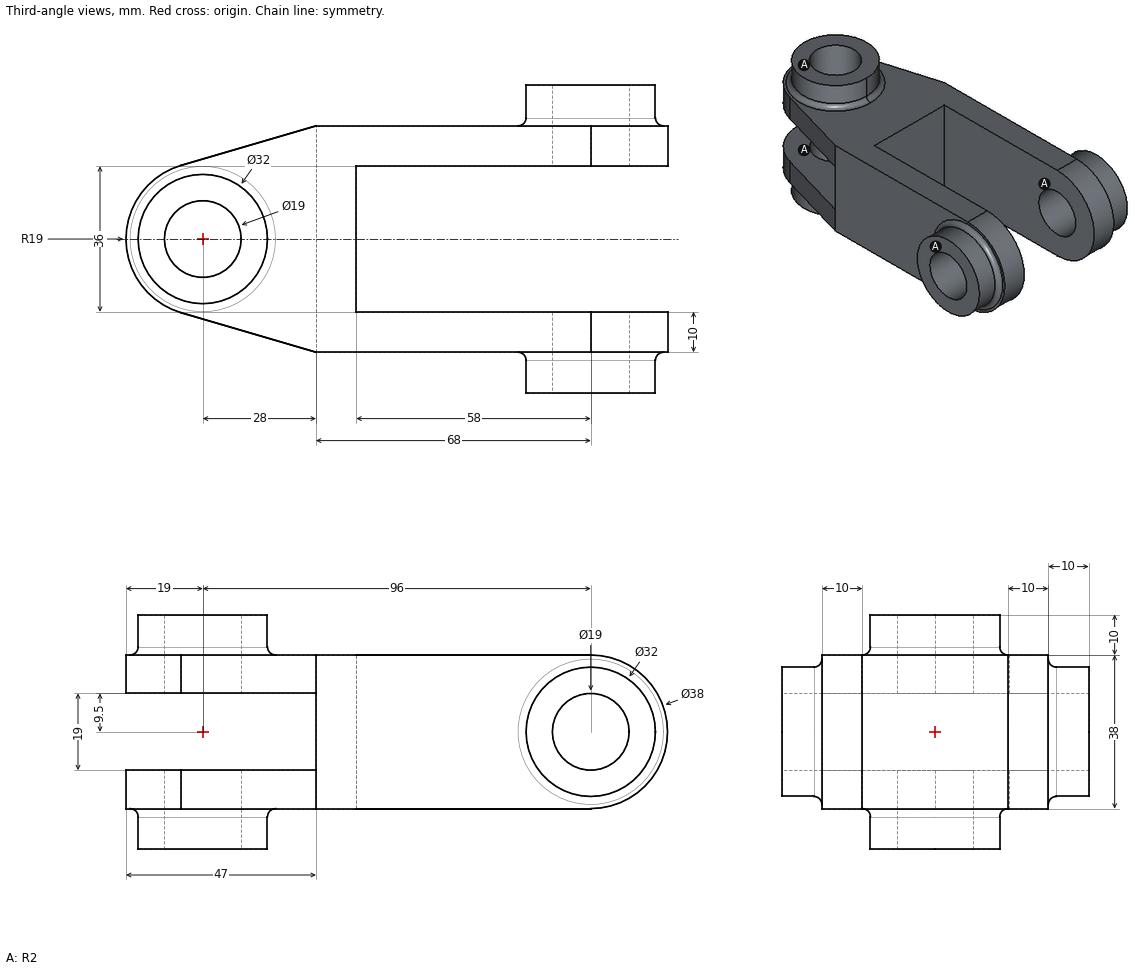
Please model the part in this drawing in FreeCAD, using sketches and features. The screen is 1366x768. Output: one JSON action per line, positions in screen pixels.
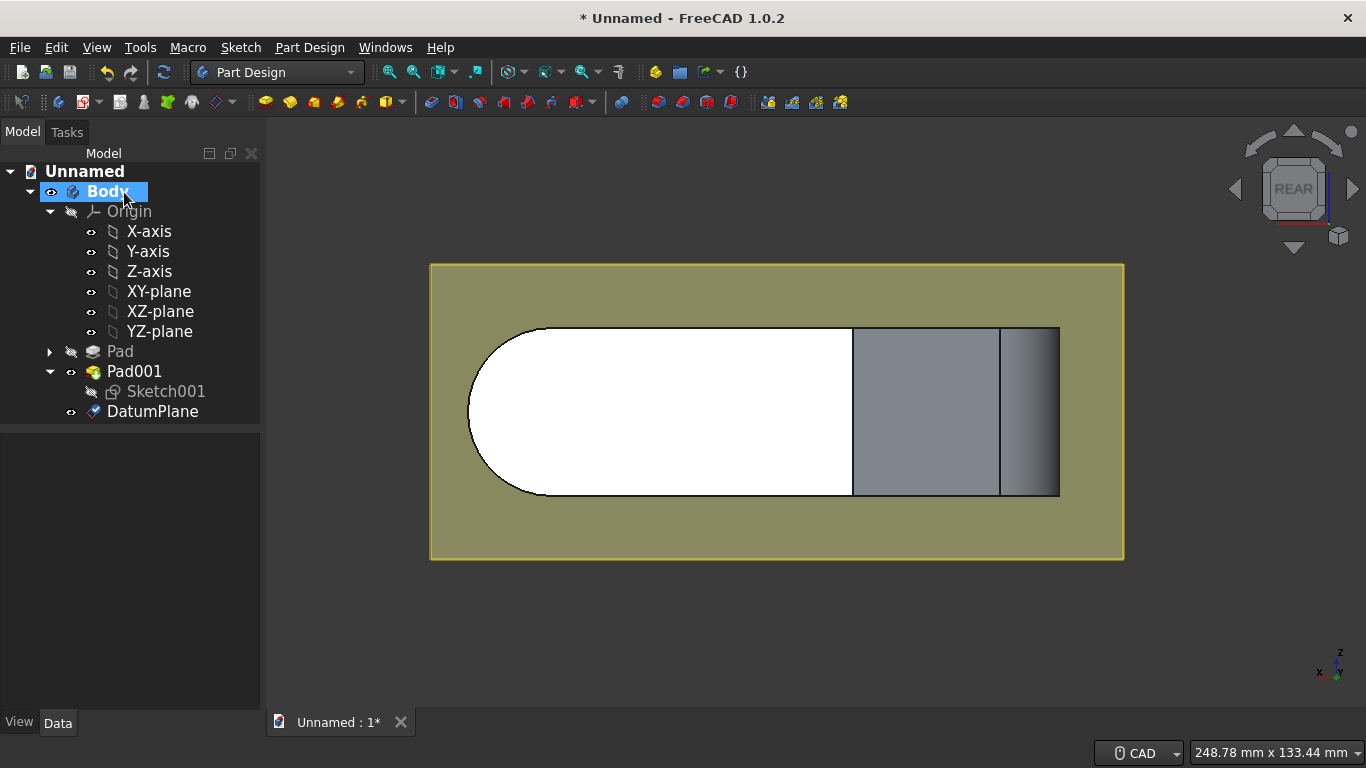
{"action": "left_click", "coordinate": [116, 412]}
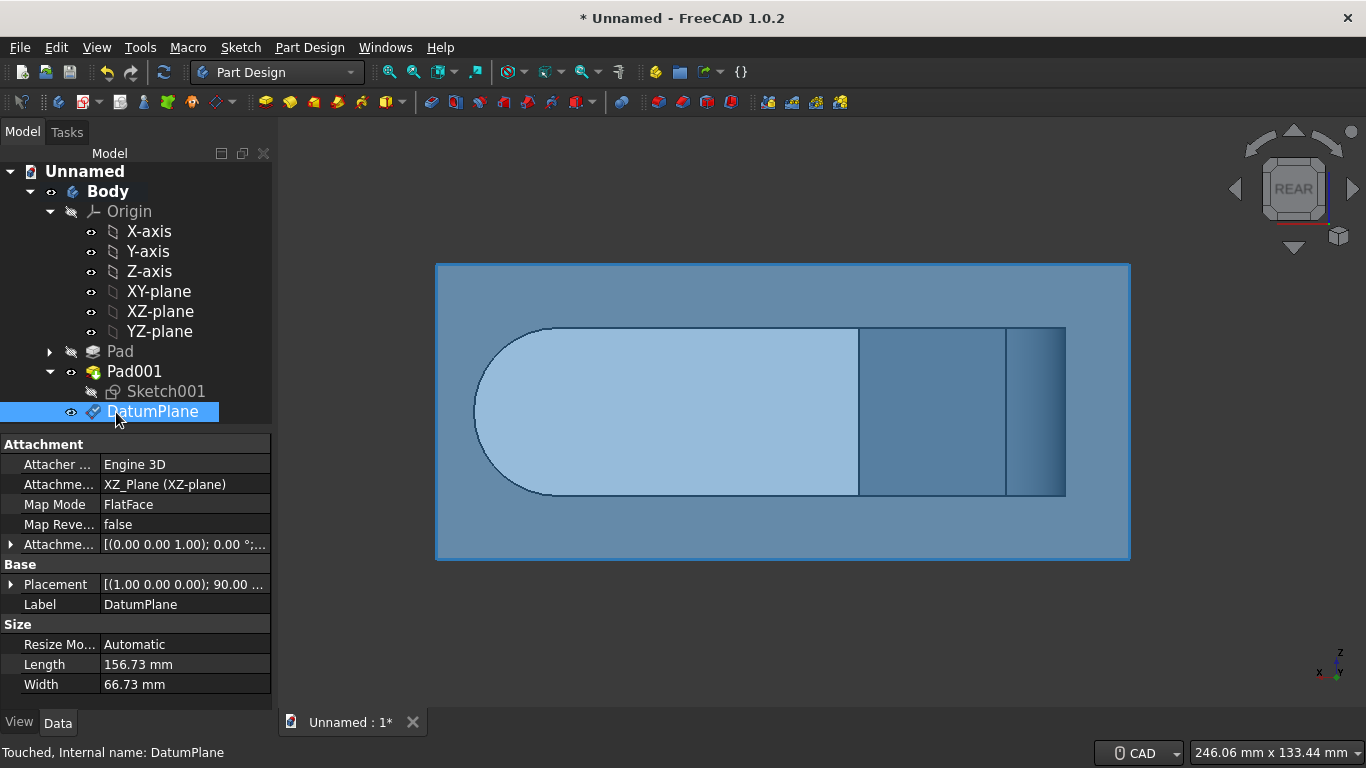
{"action": "left_click", "coordinate": [84, 102]}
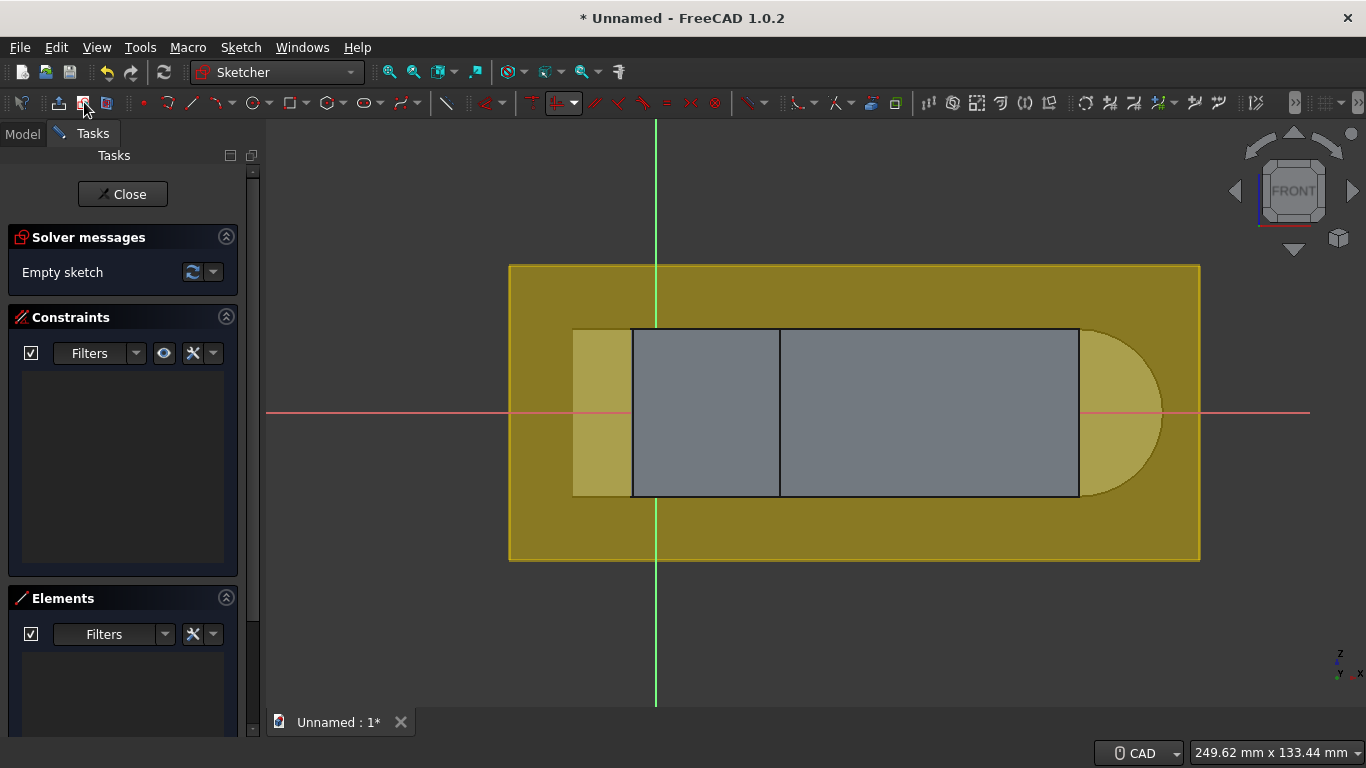
{"action": "left_click", "coordinate": [108, 104]}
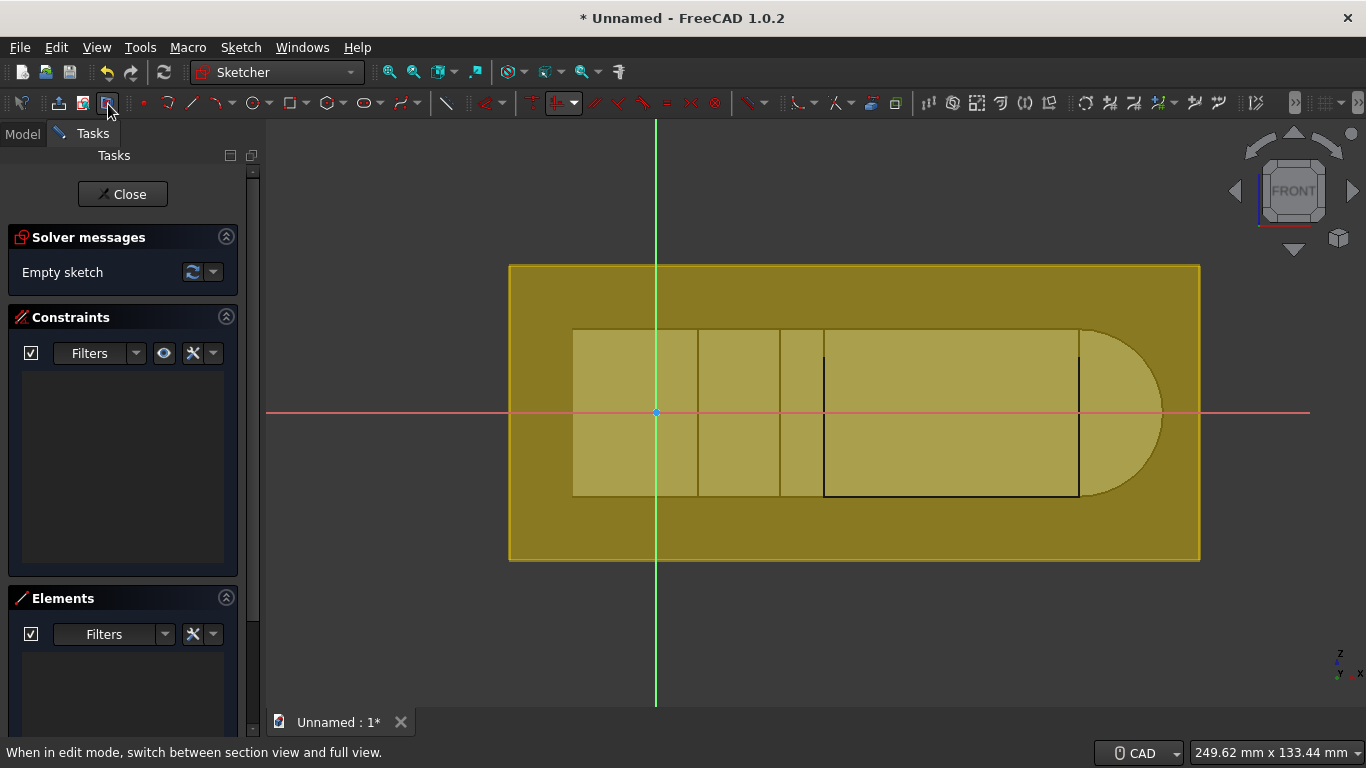
{"action": "scroll", "coordinate": [1201, 413], "scroll_direction": "up", "scroll_amount": 4}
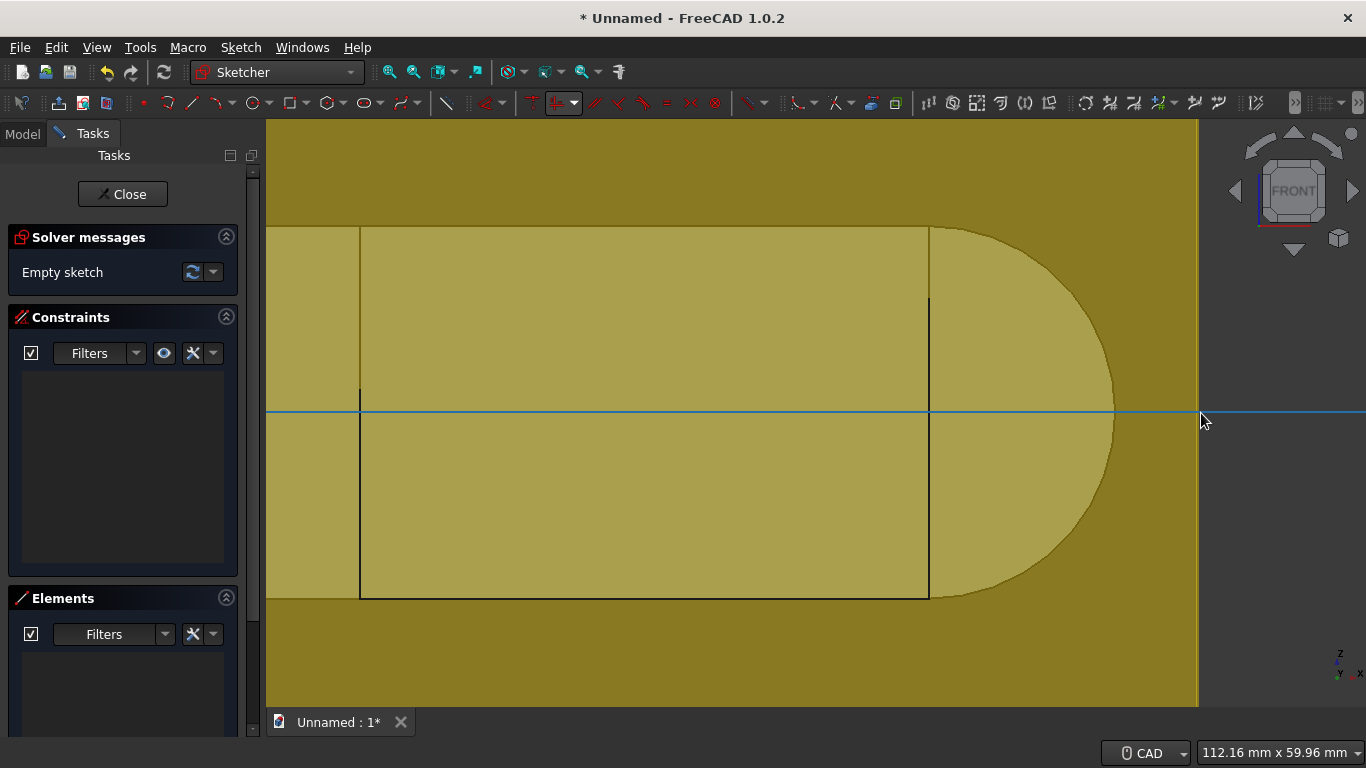
{"action": "left_click", "coordinate": [254, 104]}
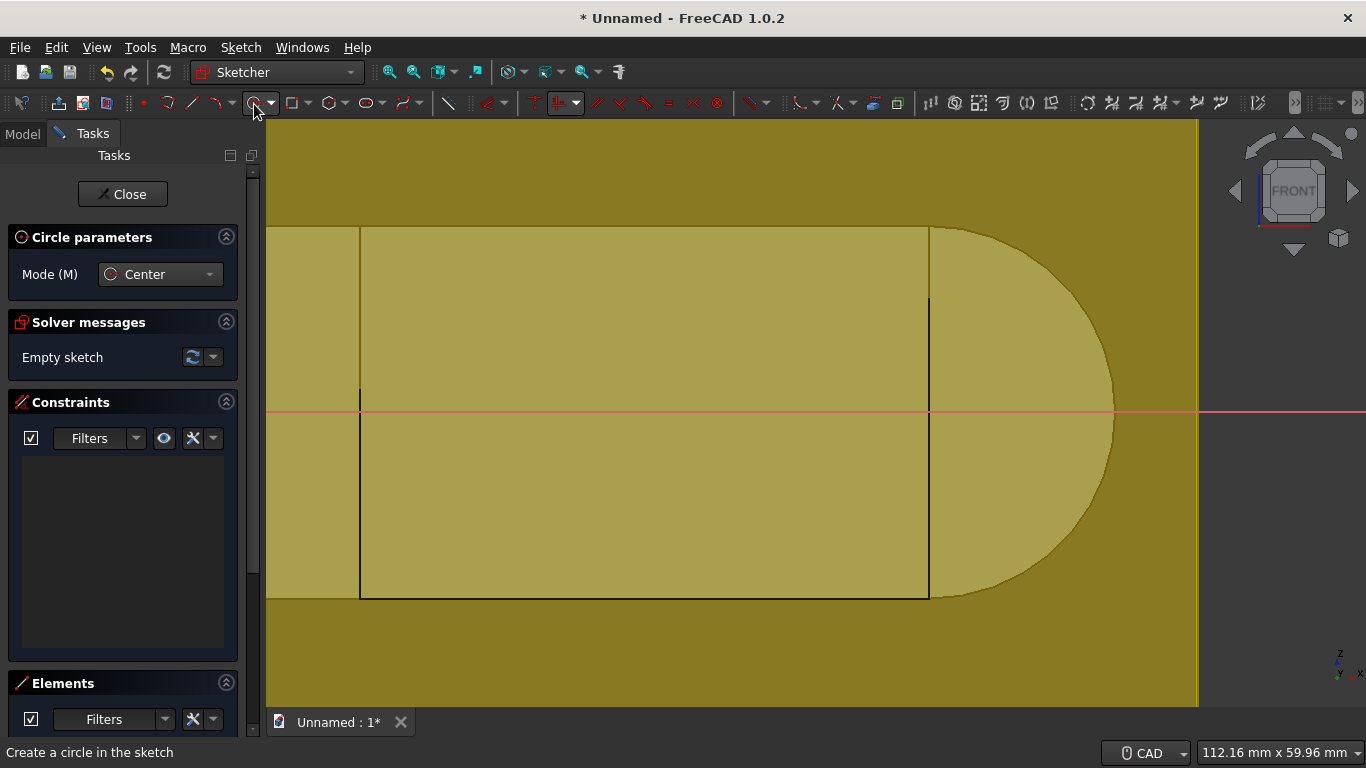
{"action": "left_click", "coordinate": [929, 412]}
{"action": "left_click", "coordinate": [1061, 281]}
{"action": "key", "text": "Escape"}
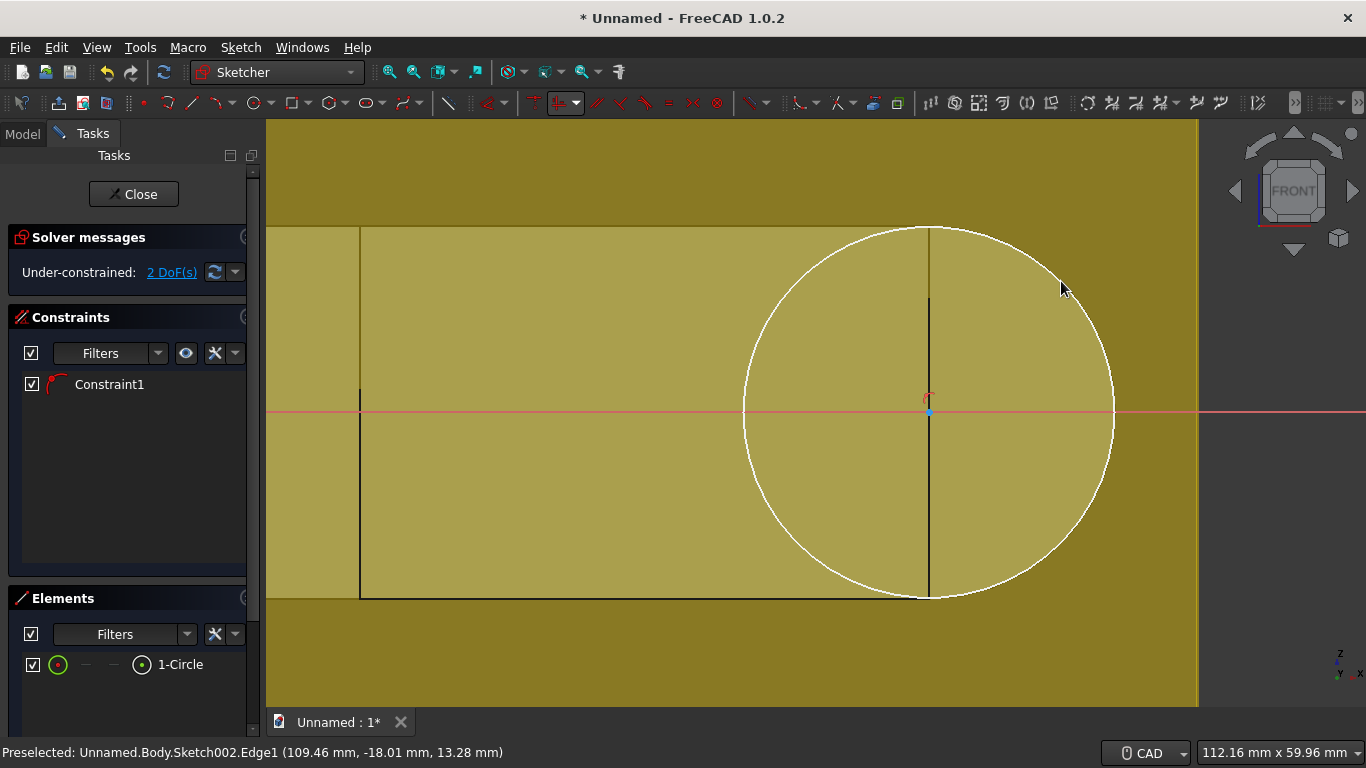
{"action": "left_click", "coordinate": [488, 104]}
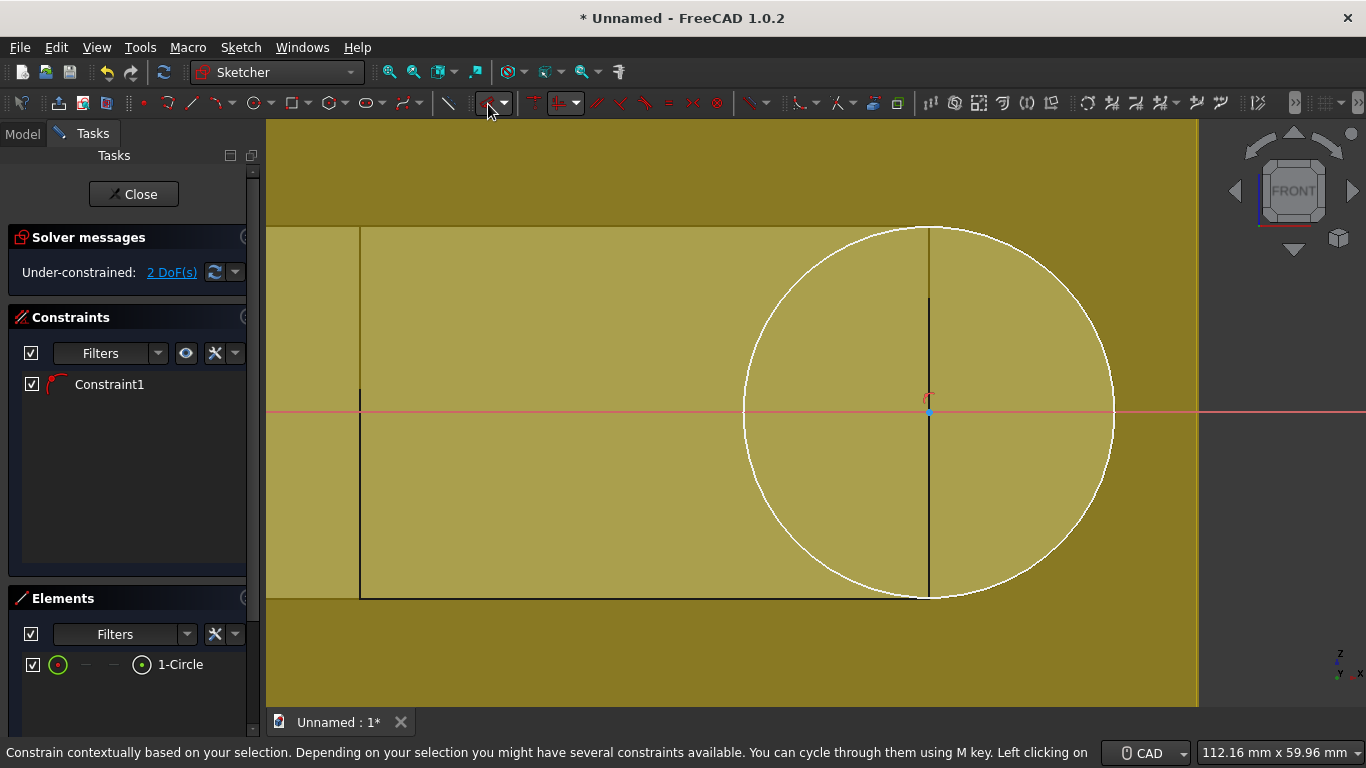
{"action": "left_click", "coordinate": [1060, 281]}
{"action": "left_click", "coordinate": [1083, 258]}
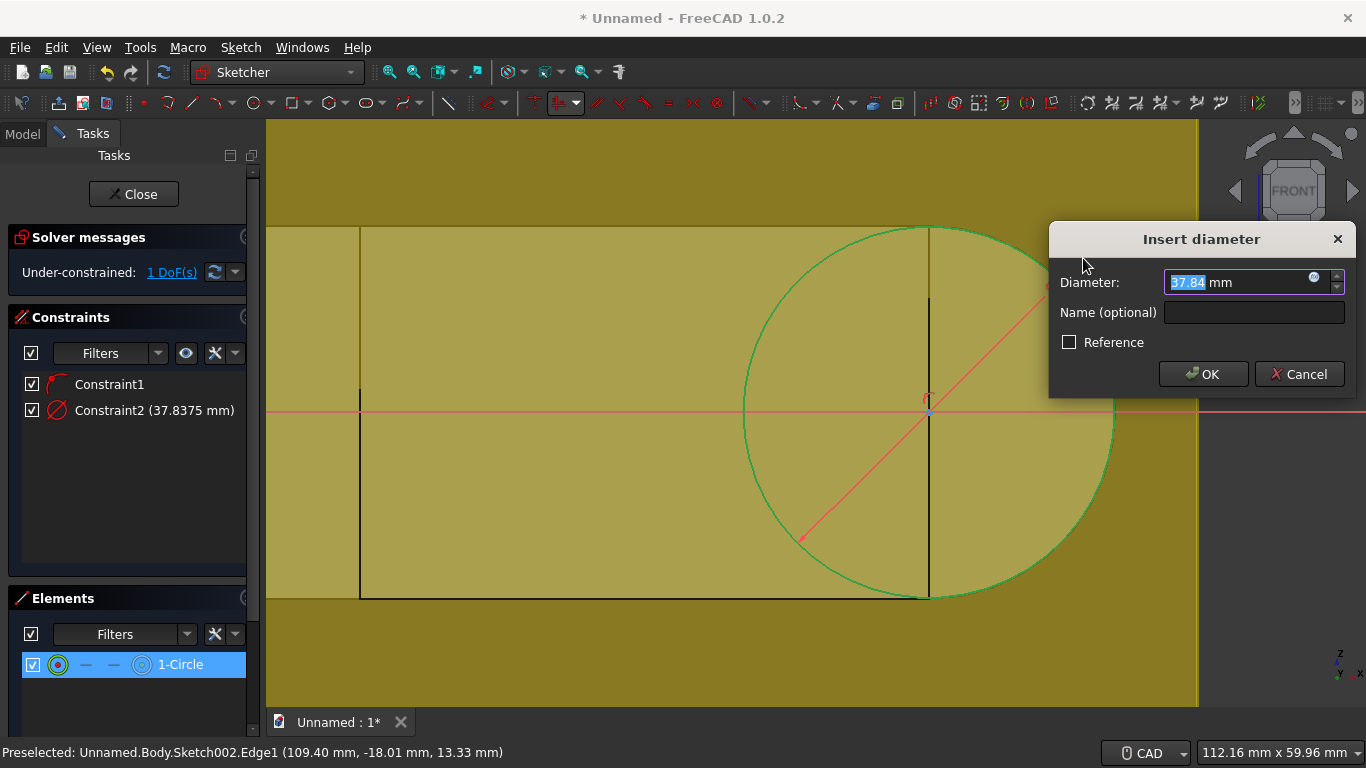
{"action": "type", "text": "38"}
{"action": "key", "text": "Return"}